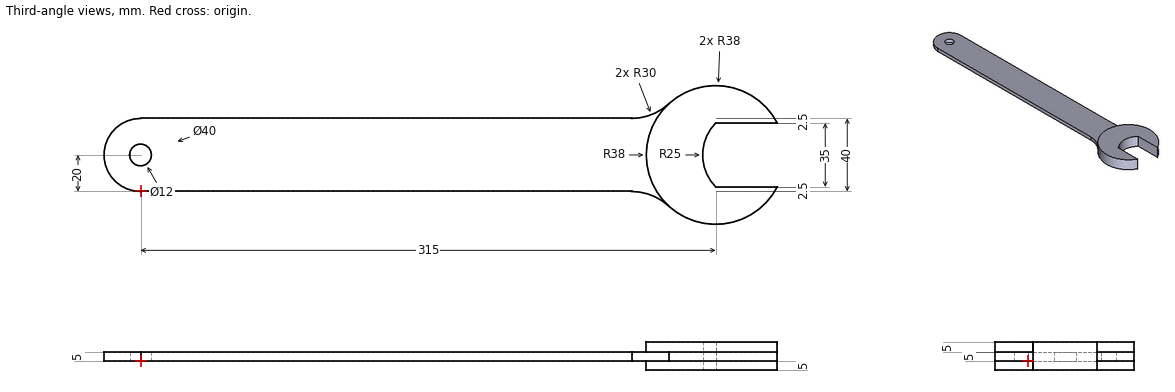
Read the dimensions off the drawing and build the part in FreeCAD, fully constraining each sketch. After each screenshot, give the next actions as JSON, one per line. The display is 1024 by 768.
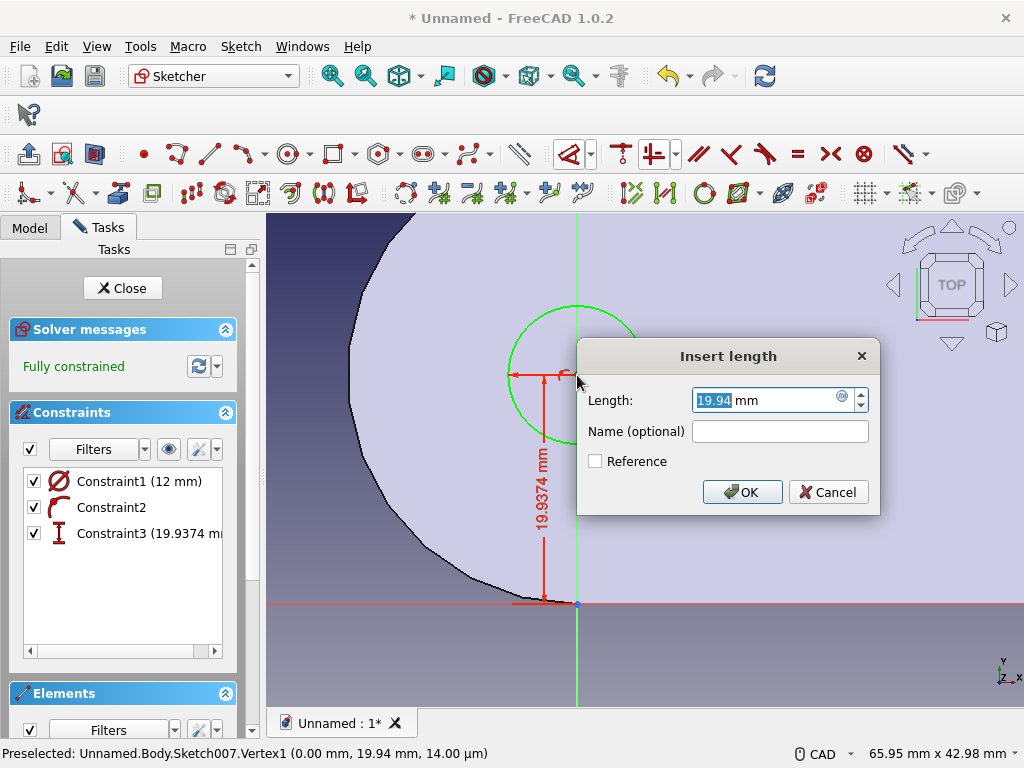
{"action": "type", "text": "20"}
{"action": "key", "text": "Return"}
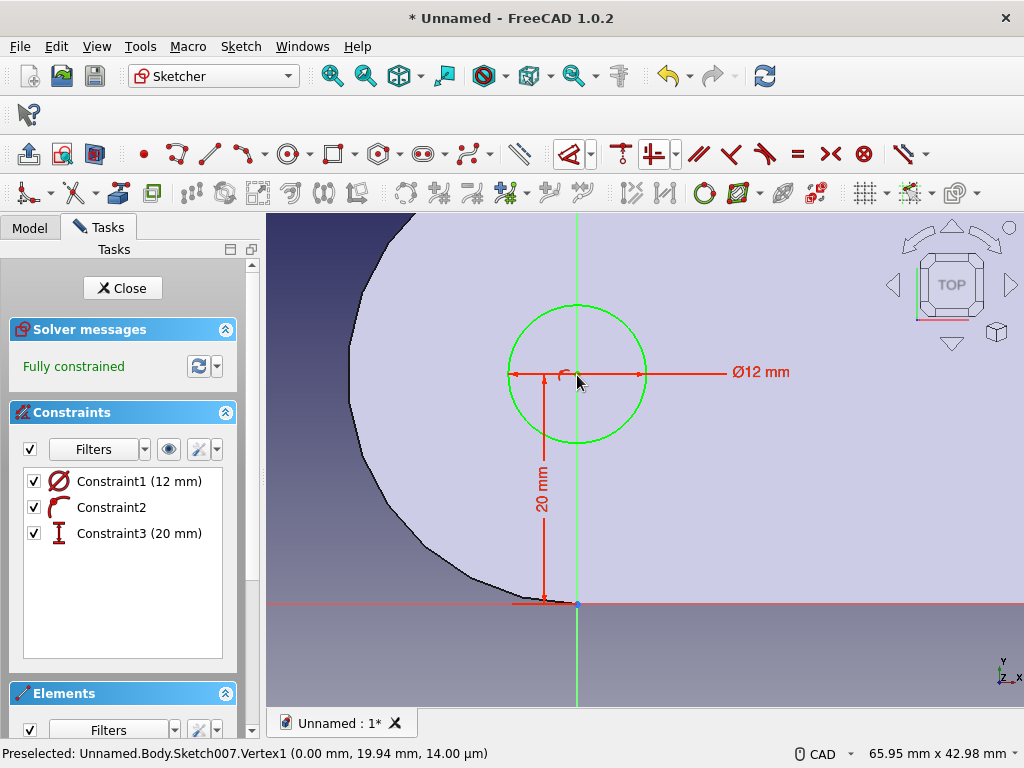
{"action": "left_click", "coordinate": [123, 288]}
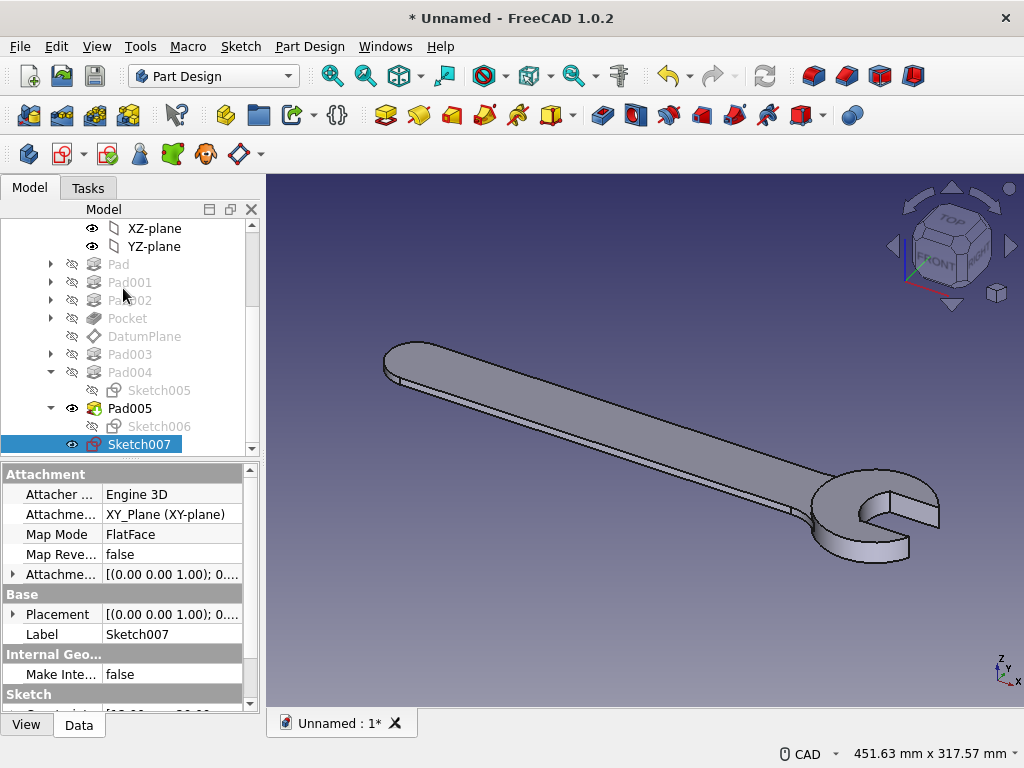
{"action": "left_click", "coordinate": [603, 116]}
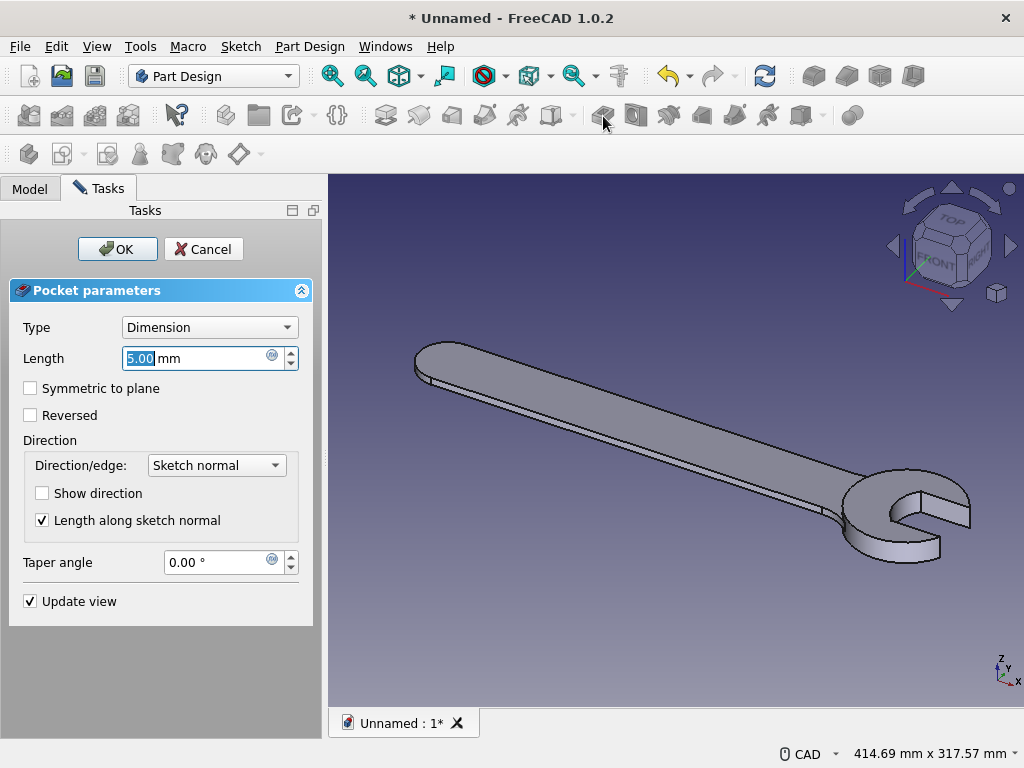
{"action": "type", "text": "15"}
{"action": "key", "text": "Tab"}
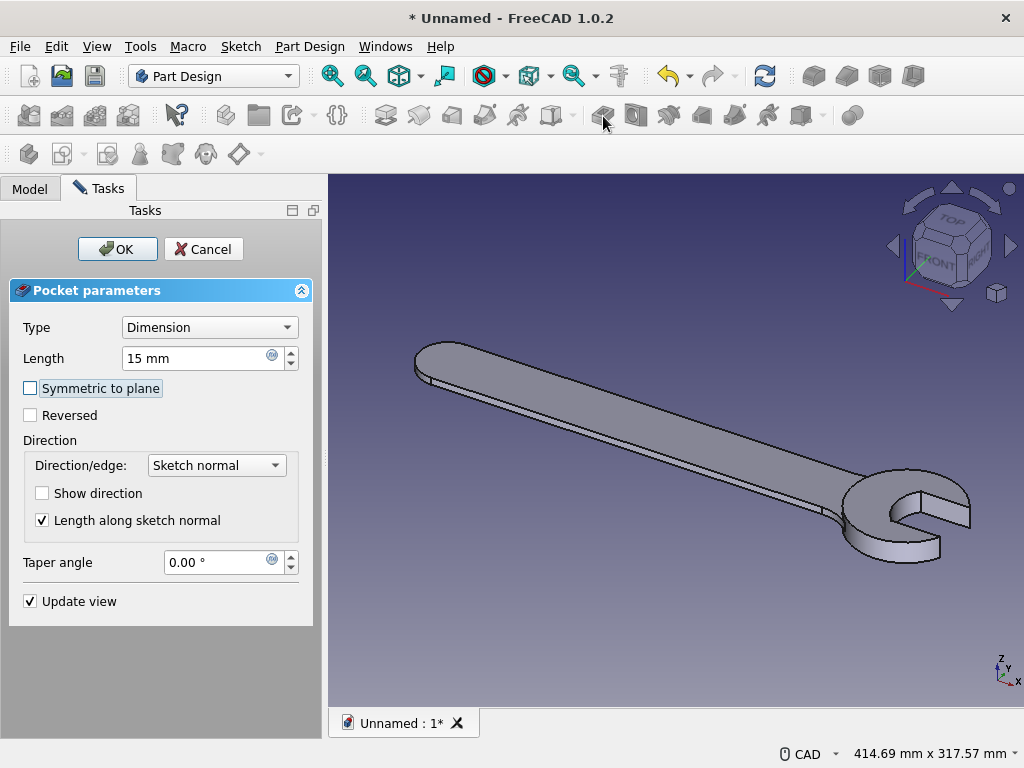
{"action": "left_click", "coordinate": [31, 415]}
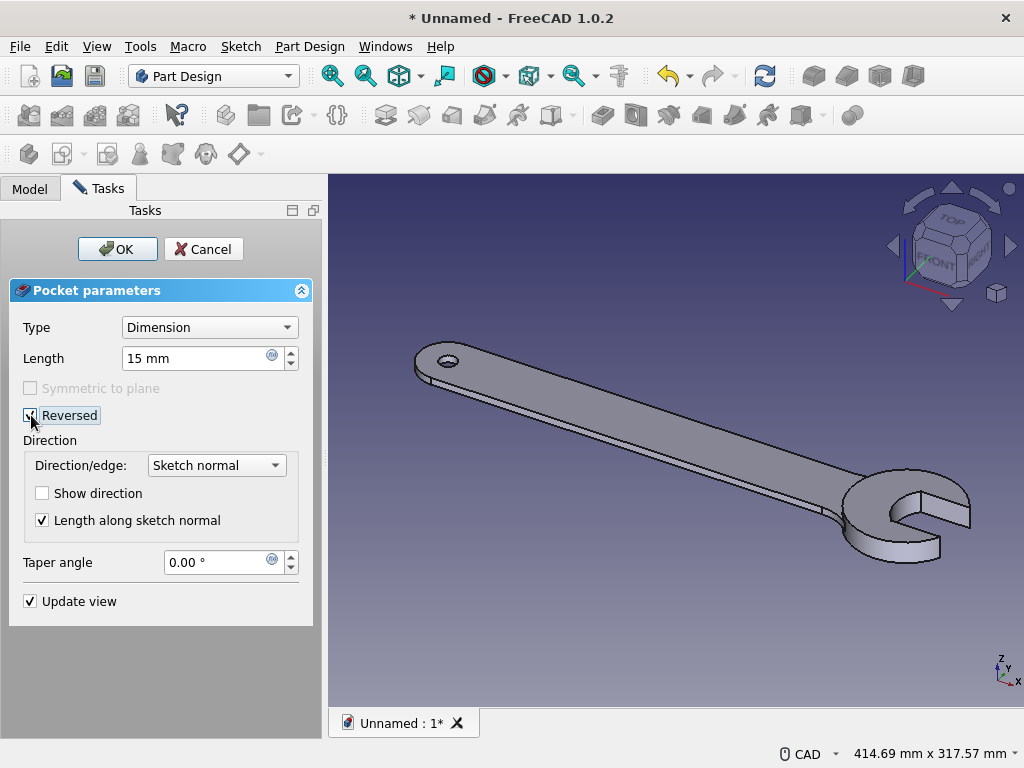
{"action": "left_click", "coordinate": [118, 249]}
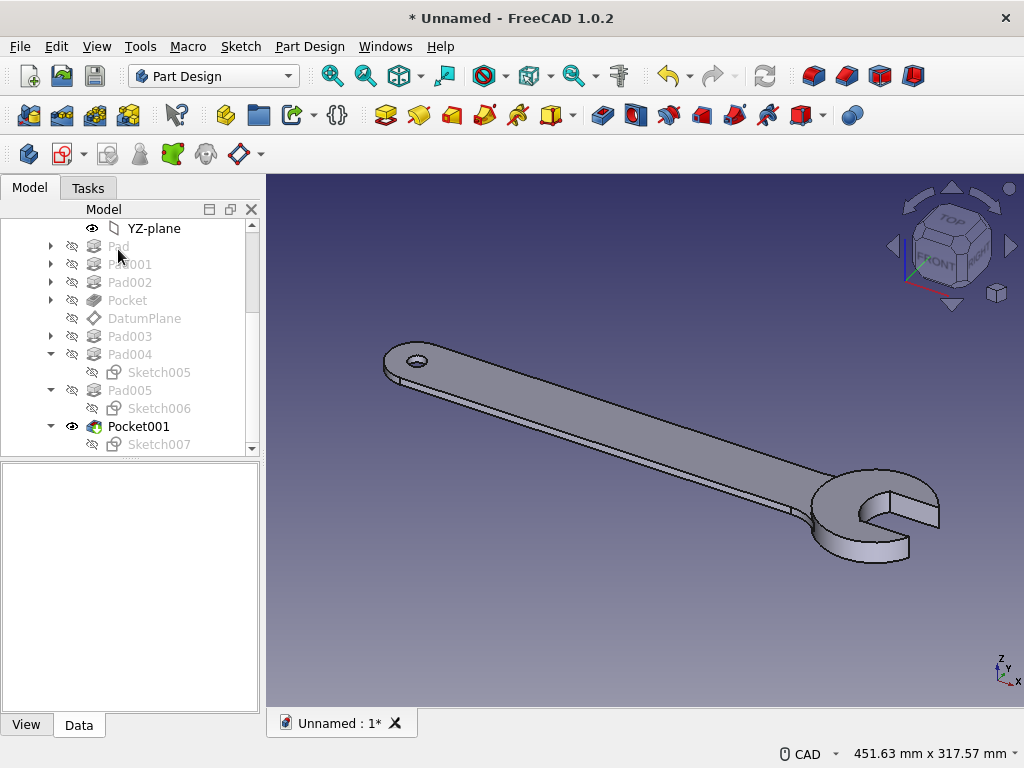
{"action": "key", "text": "0"}